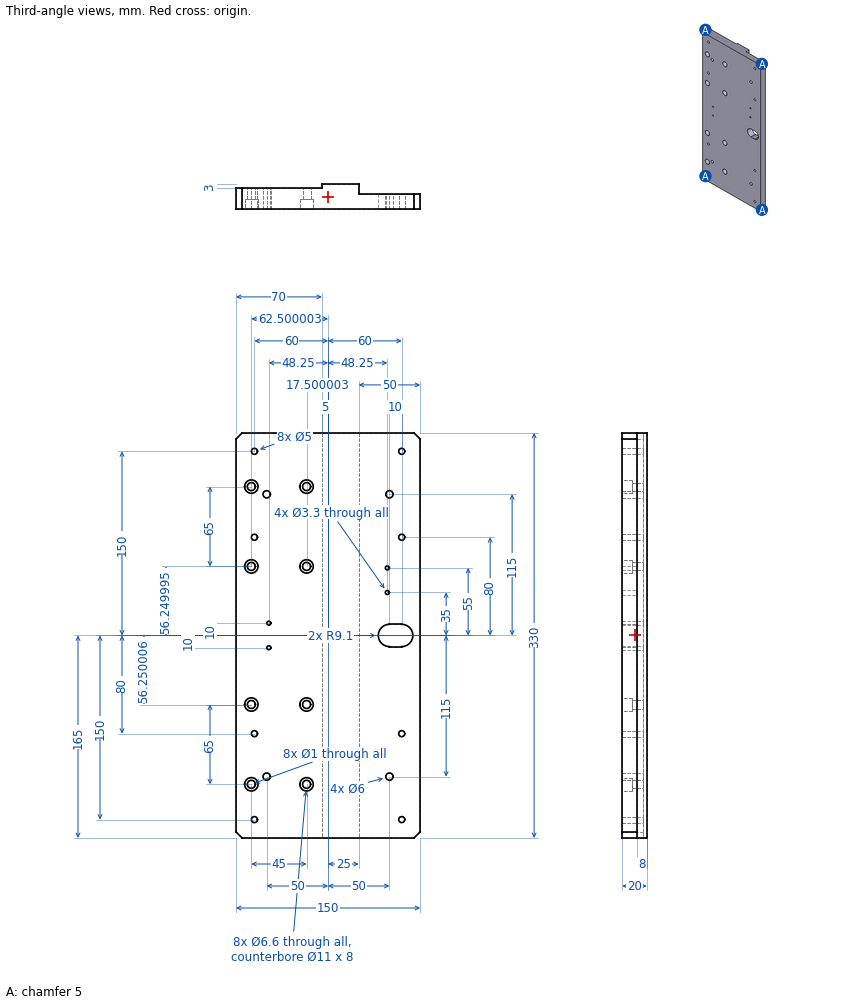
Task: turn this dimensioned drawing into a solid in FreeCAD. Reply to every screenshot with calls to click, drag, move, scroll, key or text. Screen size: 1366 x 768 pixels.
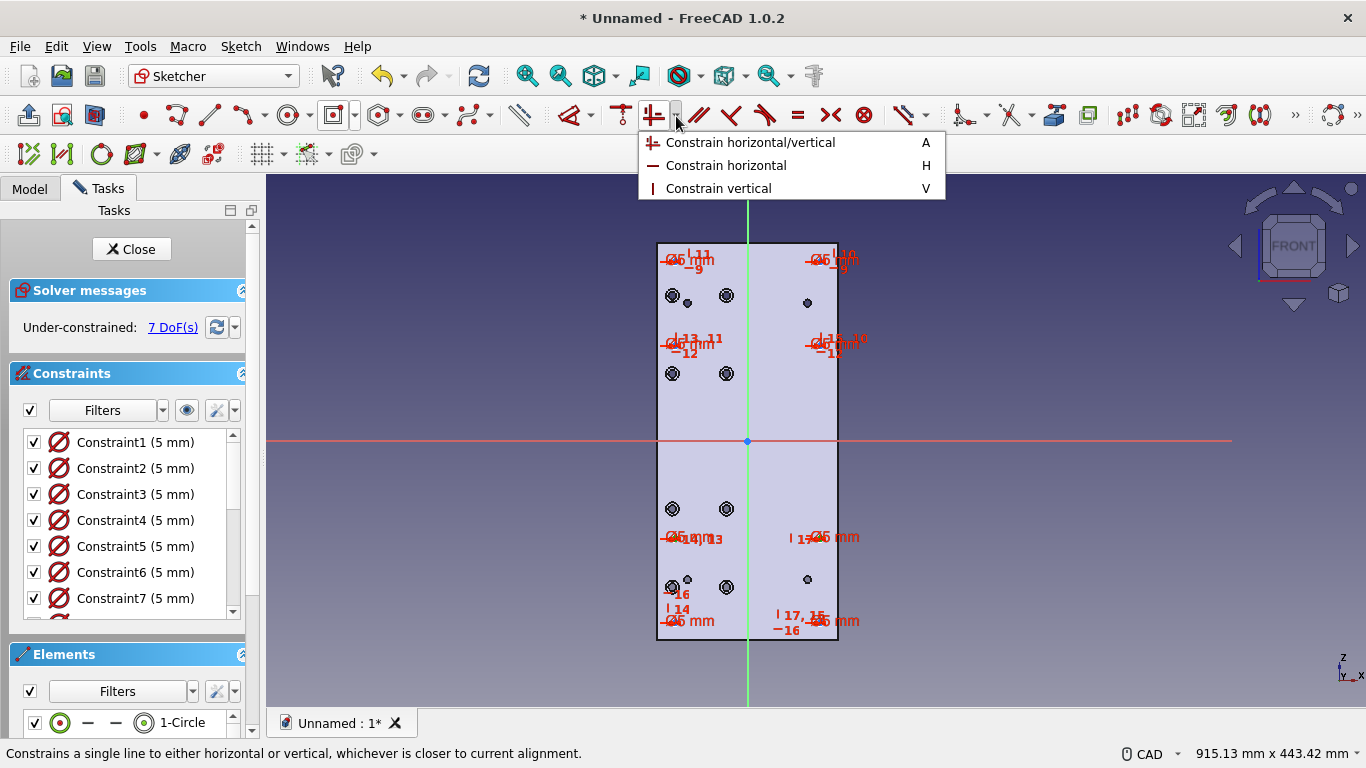
click(792, 166)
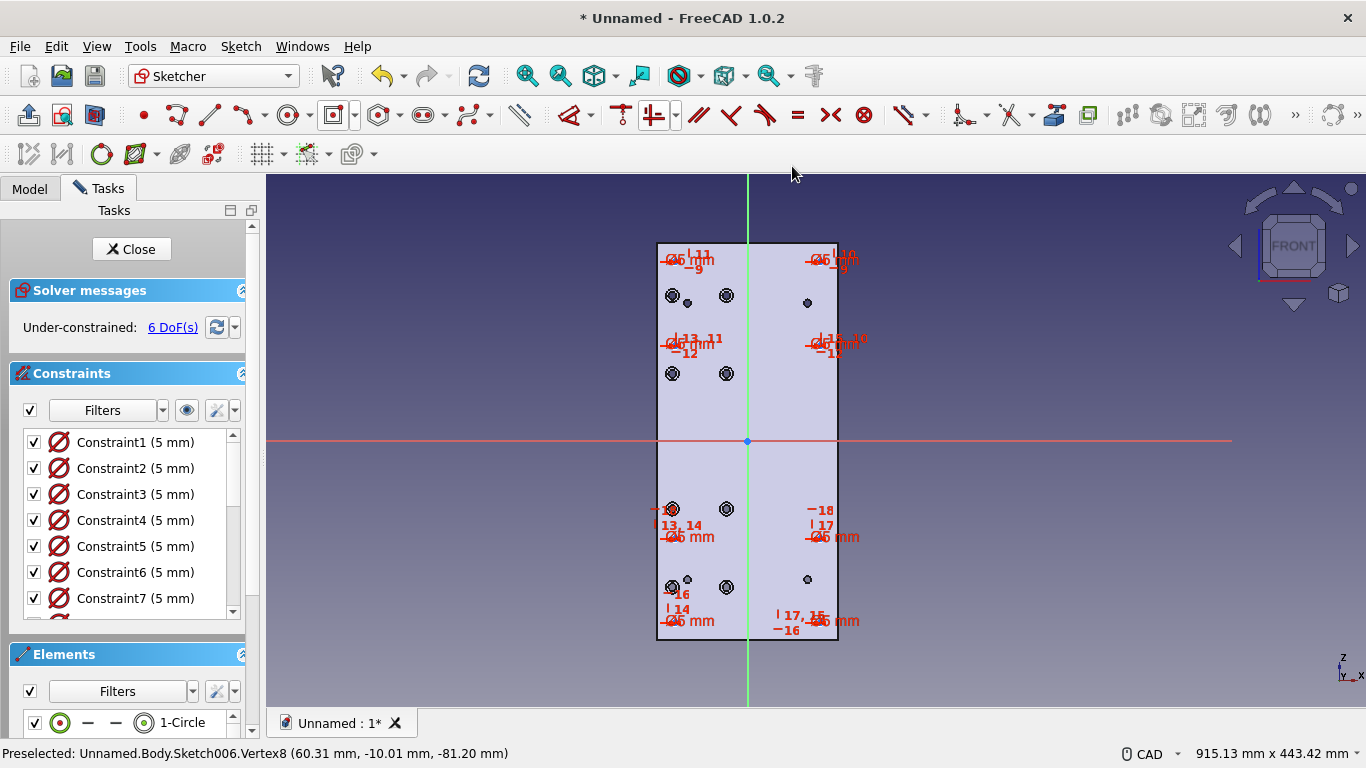
click(568, 116)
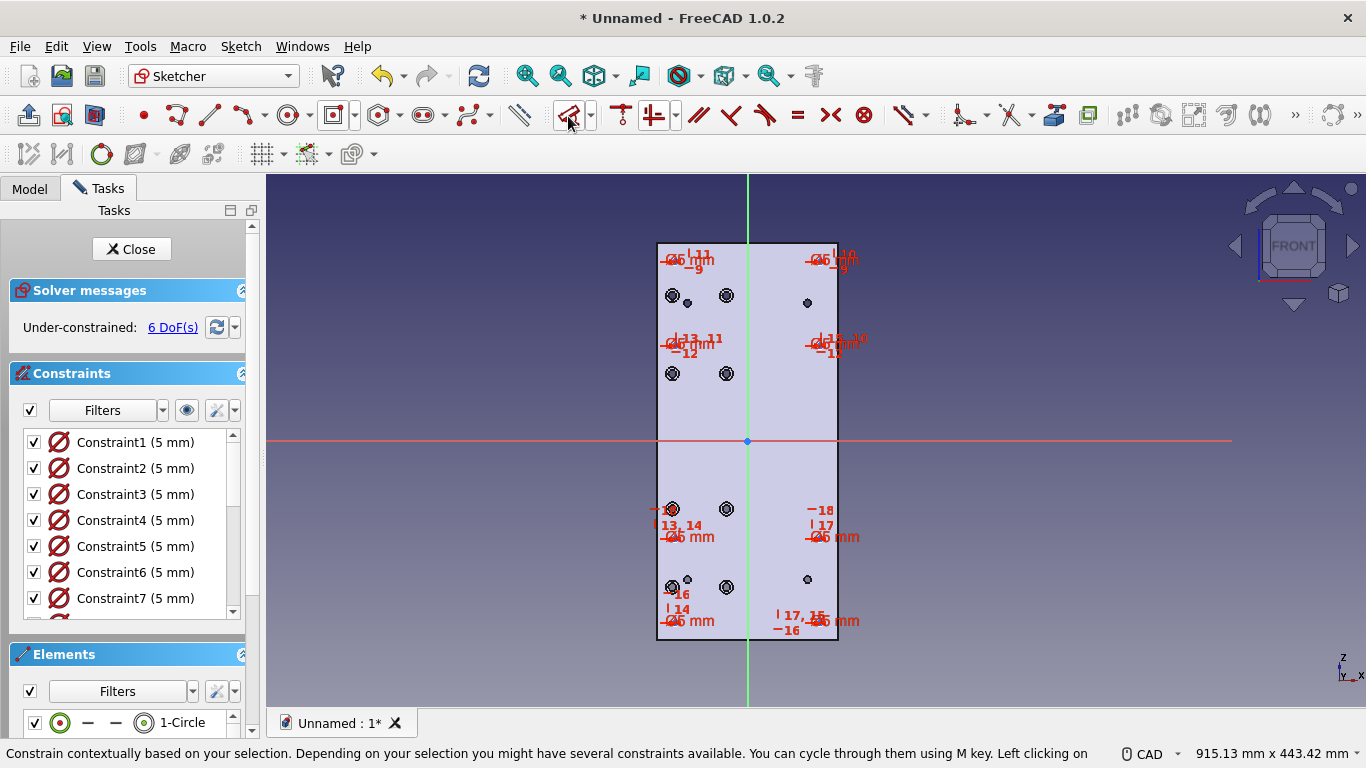
click(675, 262)
click(711, 228)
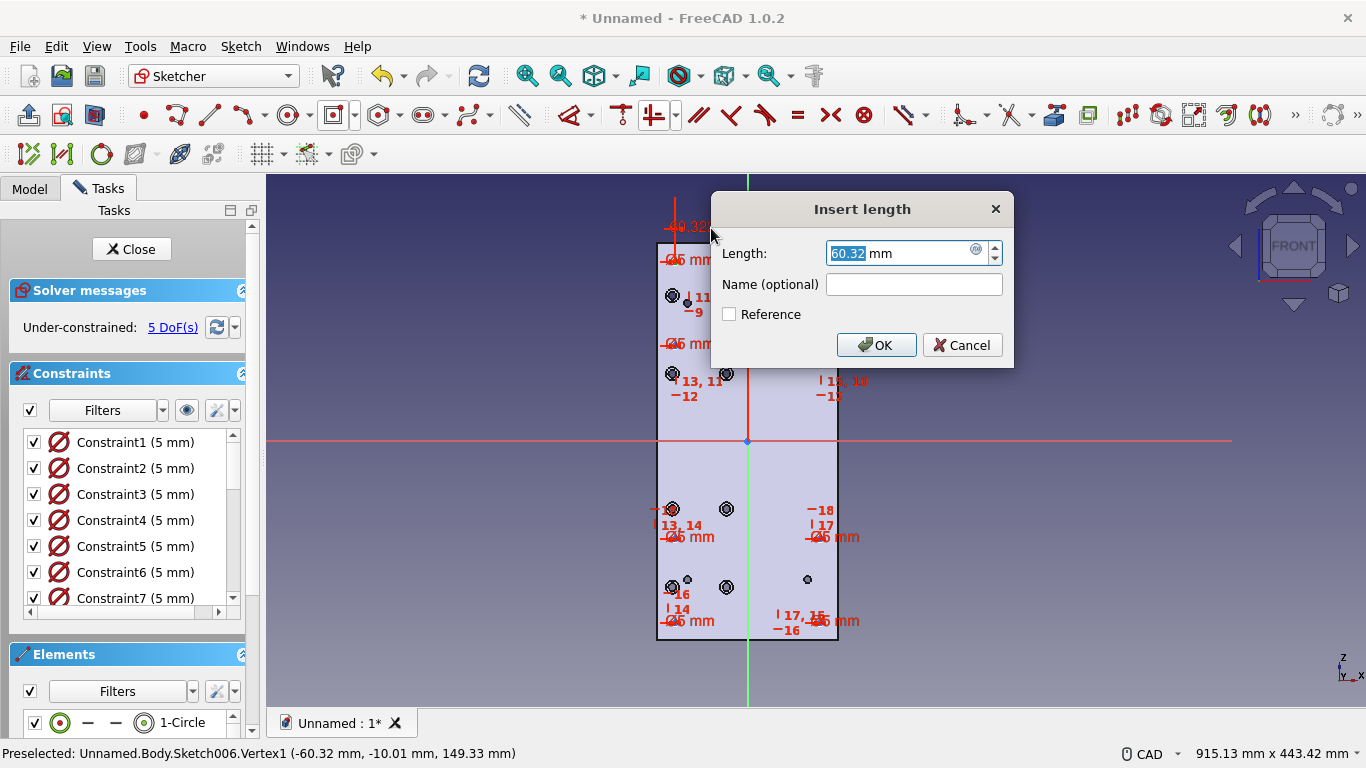
text(60)
key(Return)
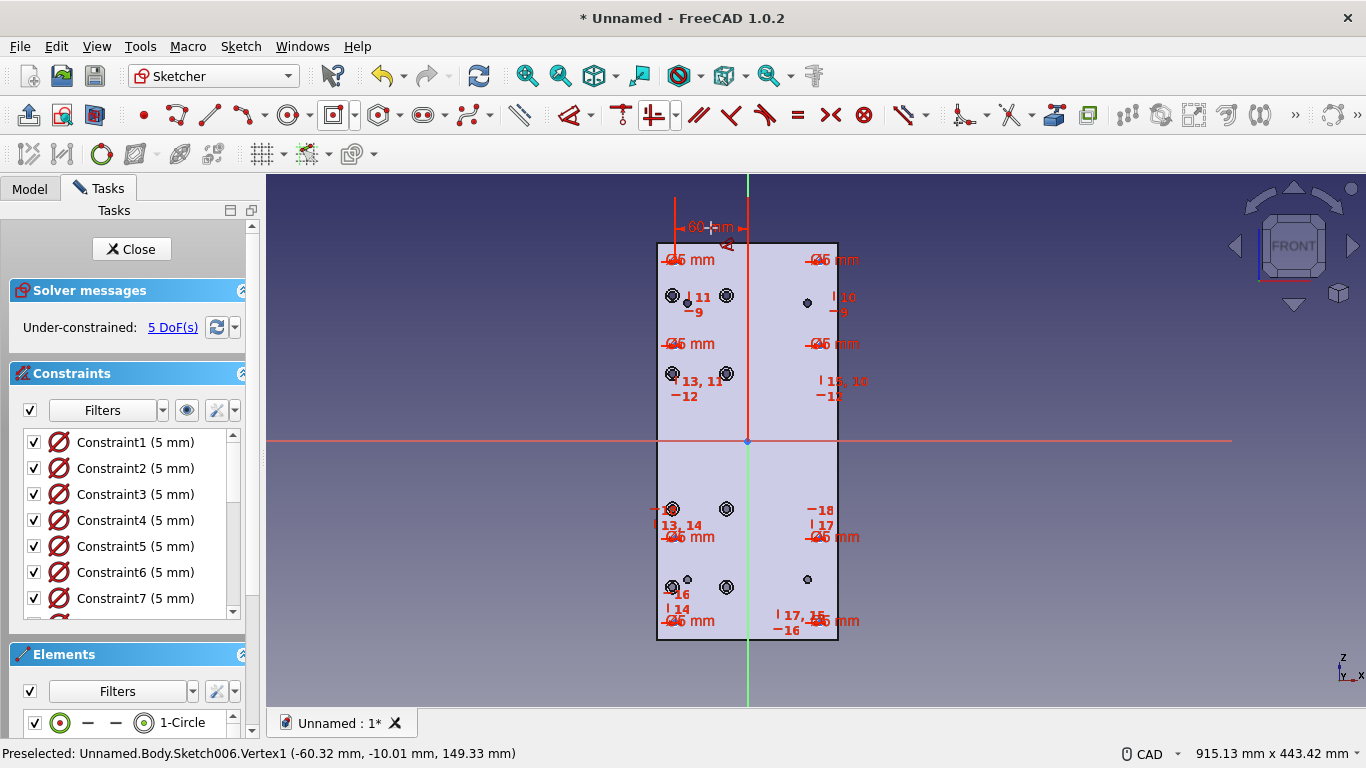
click(820, 262)
click(784, 228)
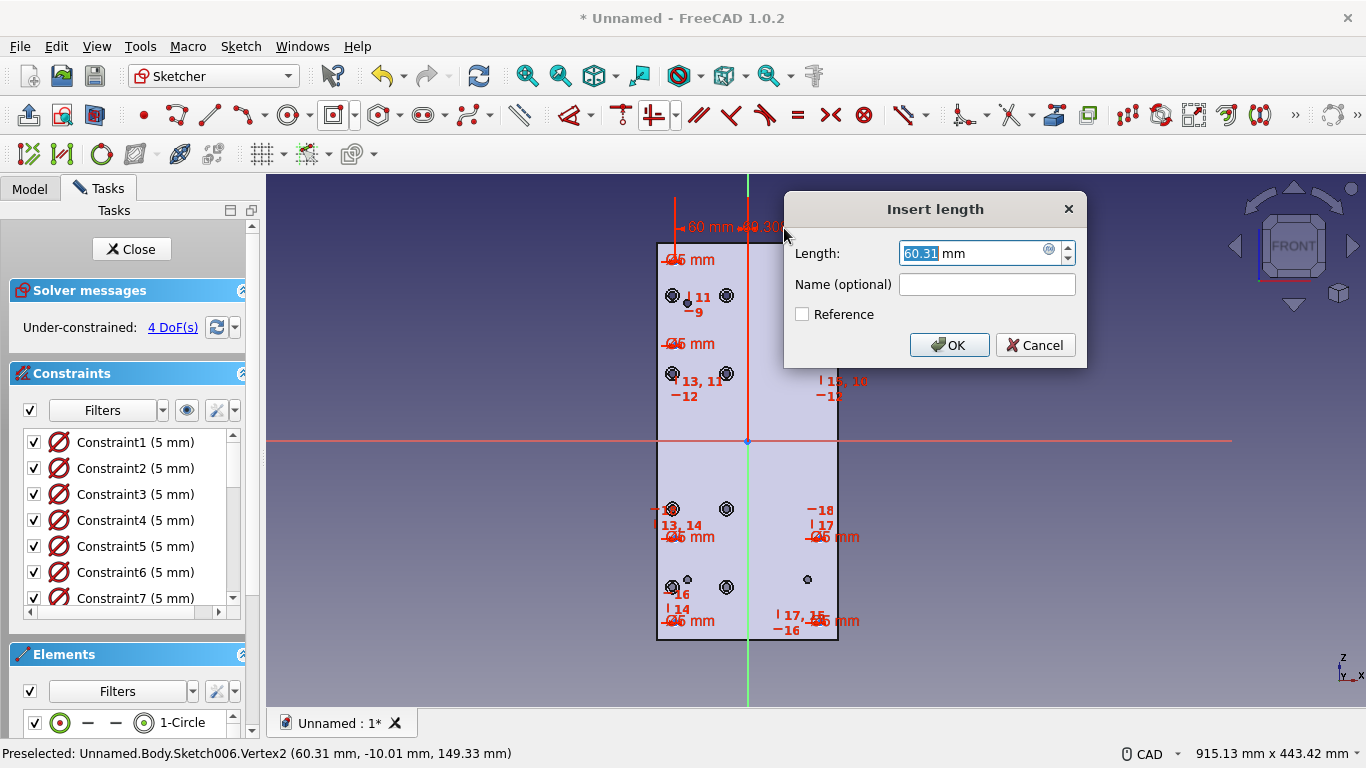
text(60)
key(Return)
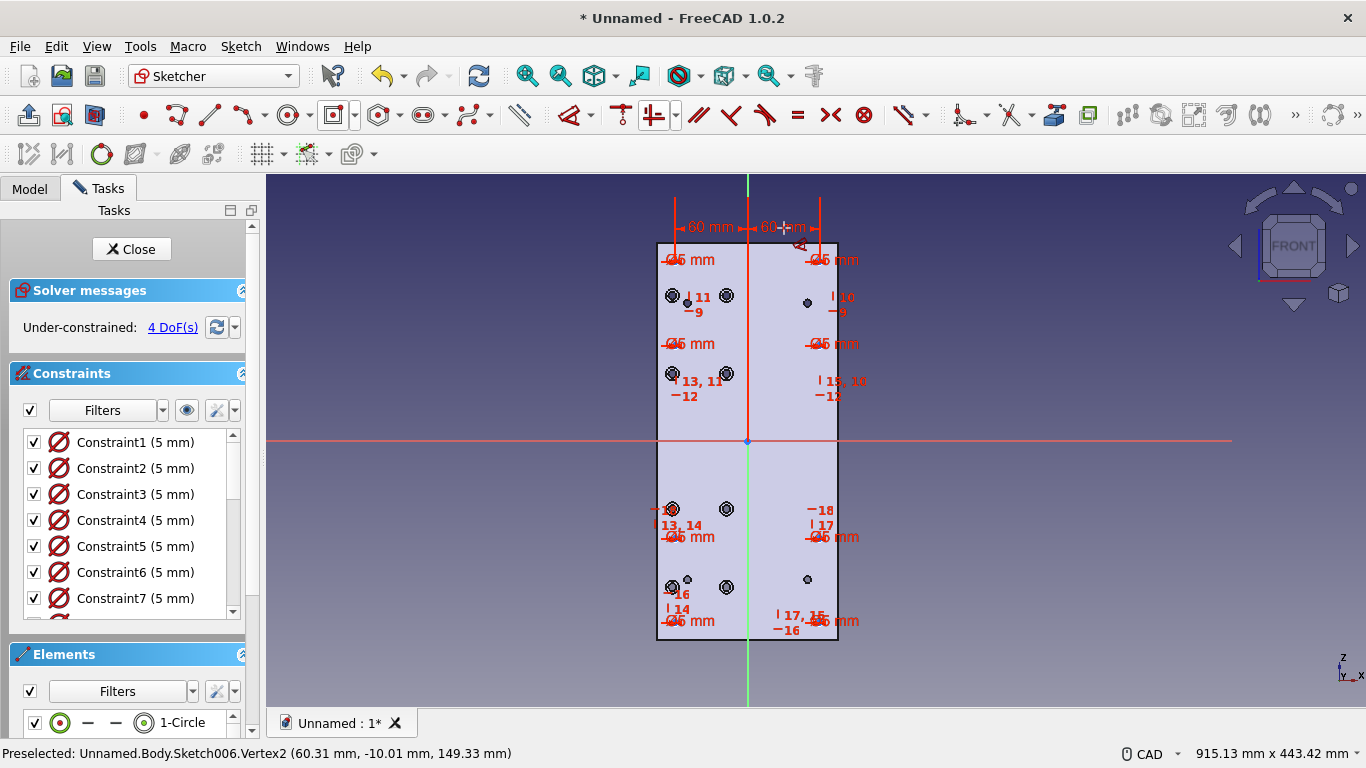
click(820, 346)
click(854, 394)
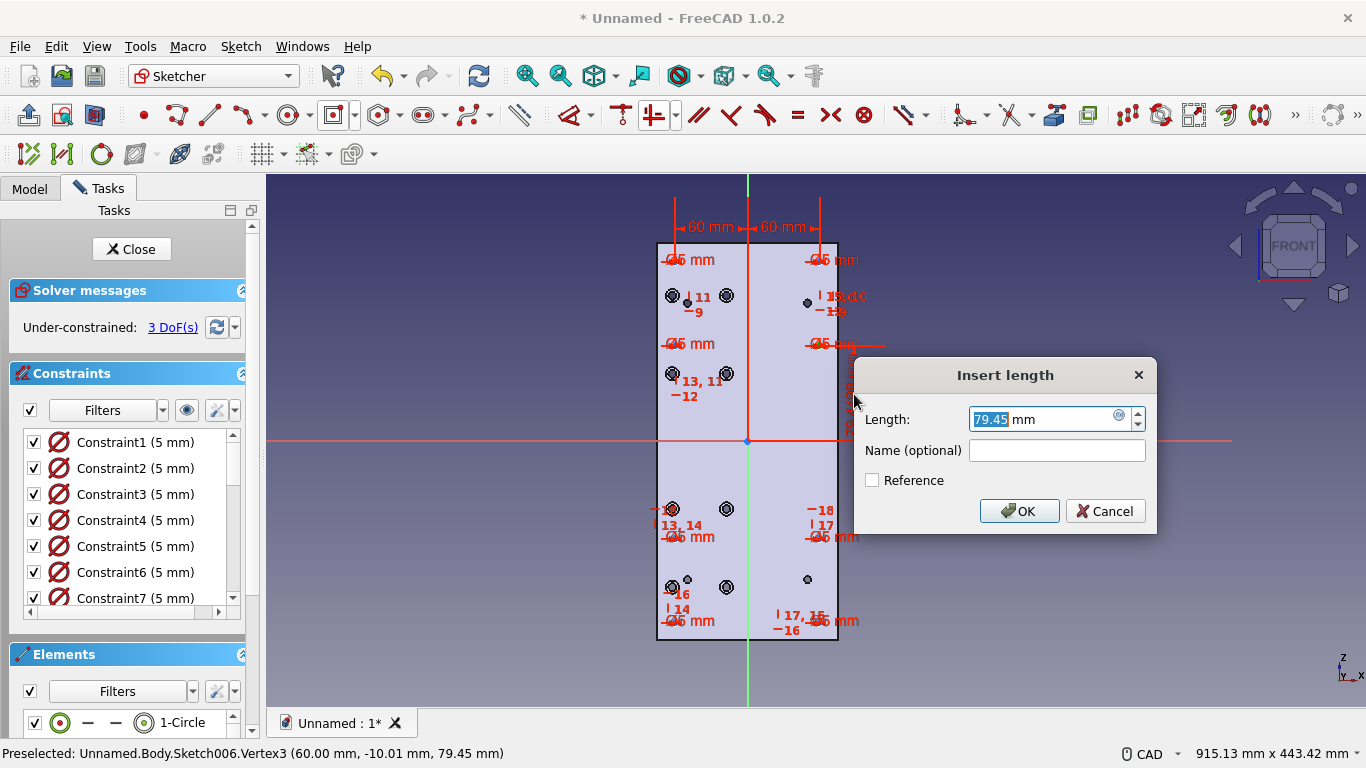
text(80)
key(Return)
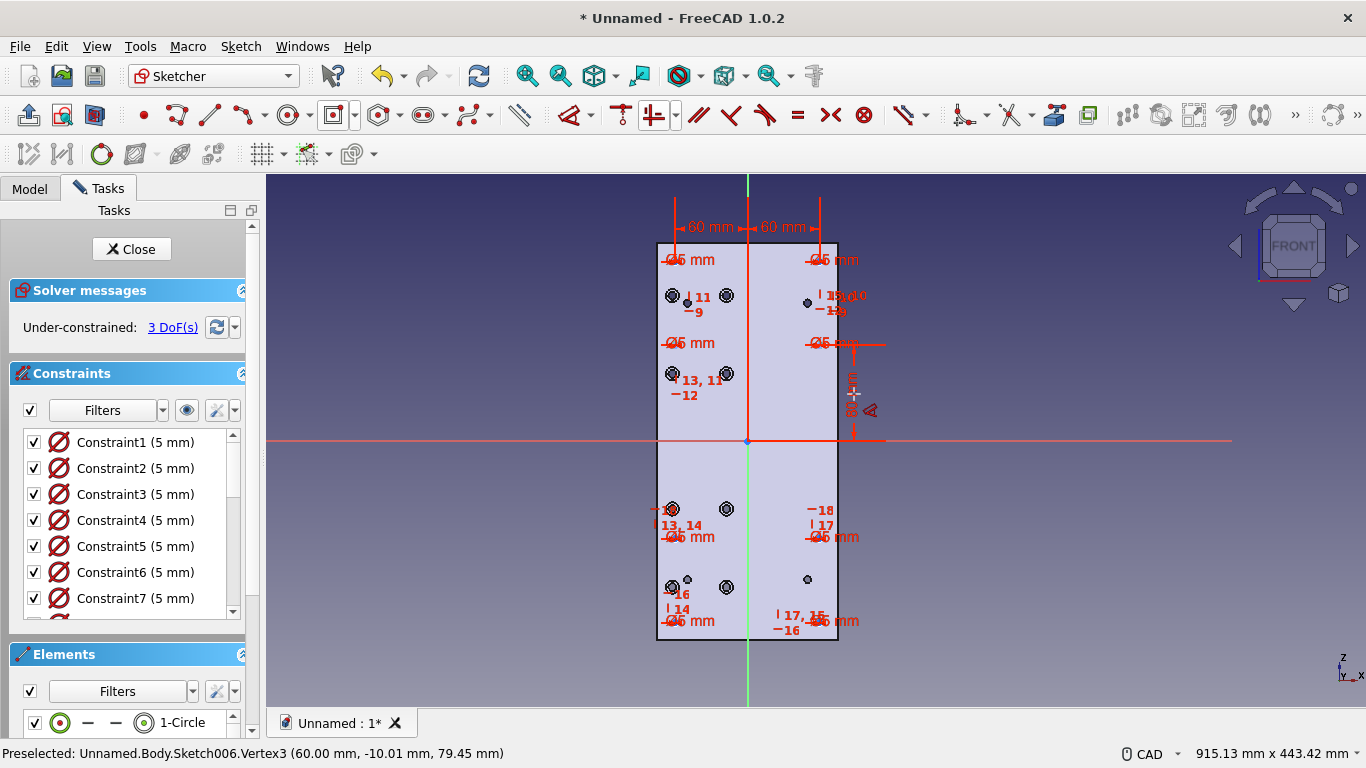
click(675, 539)
click(641, 490)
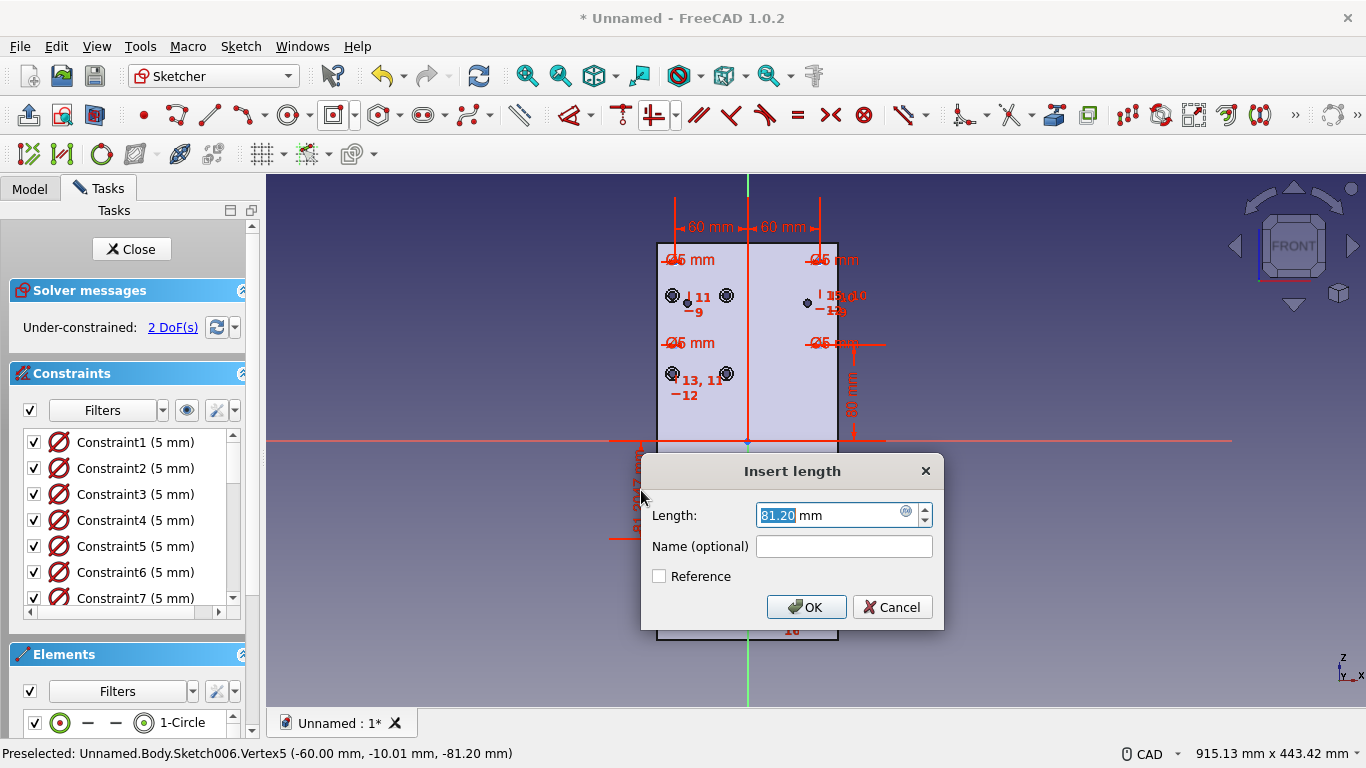
text(80)
key(Return)